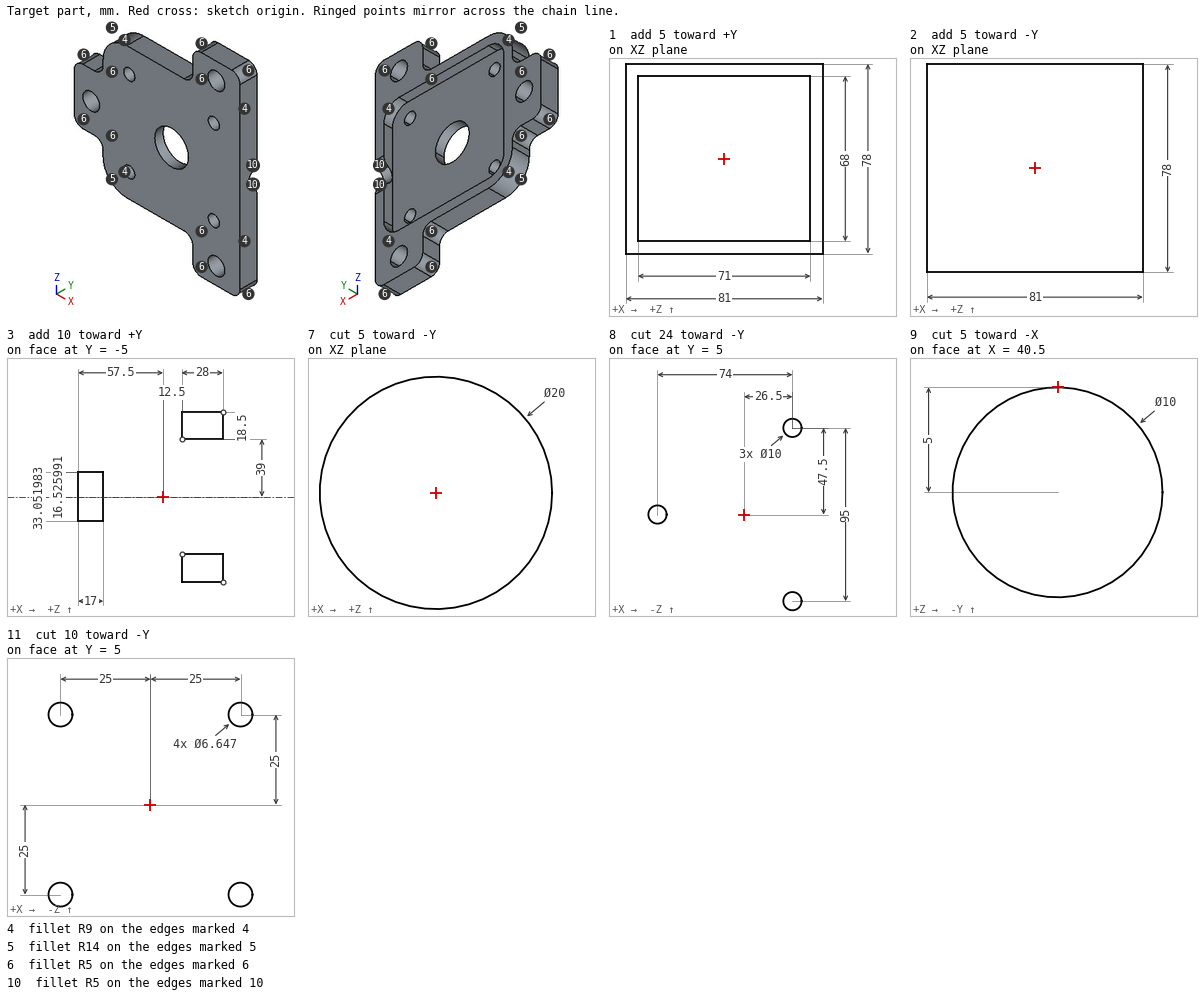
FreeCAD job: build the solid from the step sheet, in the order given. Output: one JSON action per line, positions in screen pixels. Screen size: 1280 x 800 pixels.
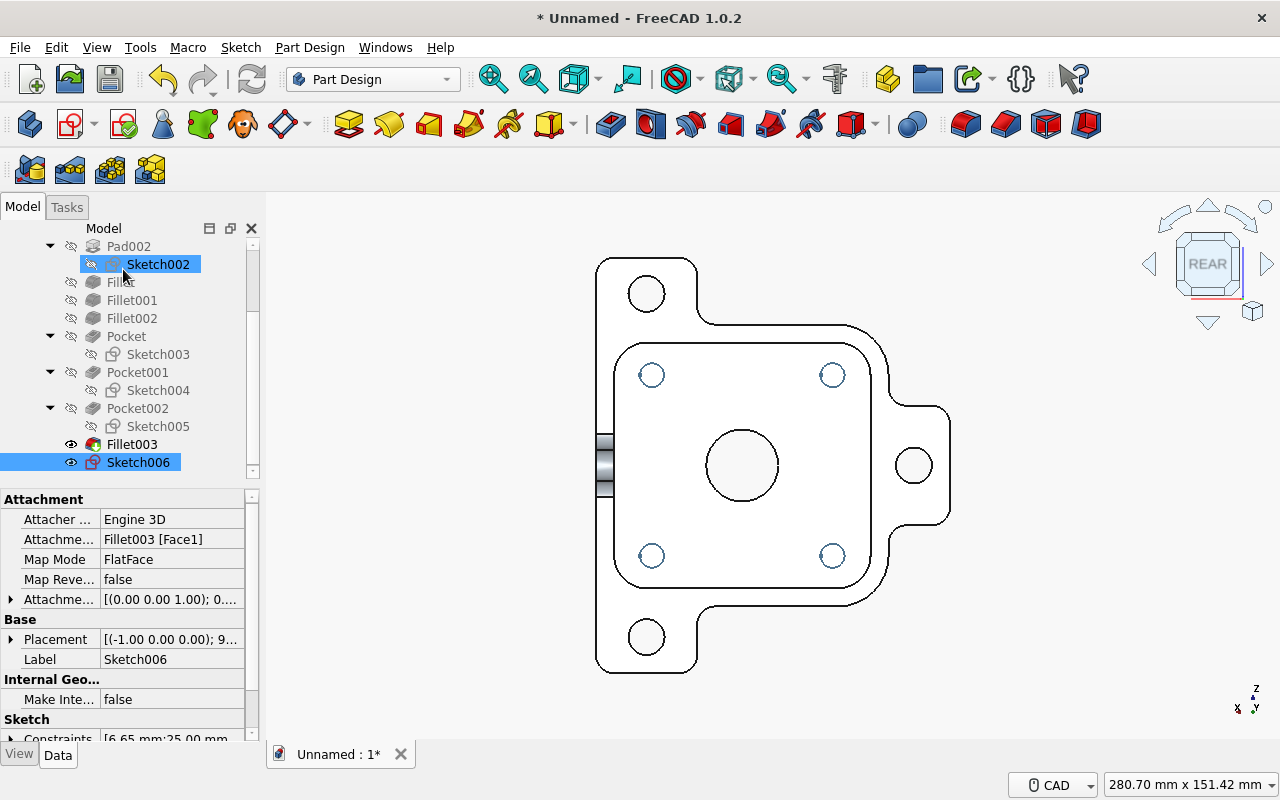
{"action": "left_click", "coordinate": [612, 124]}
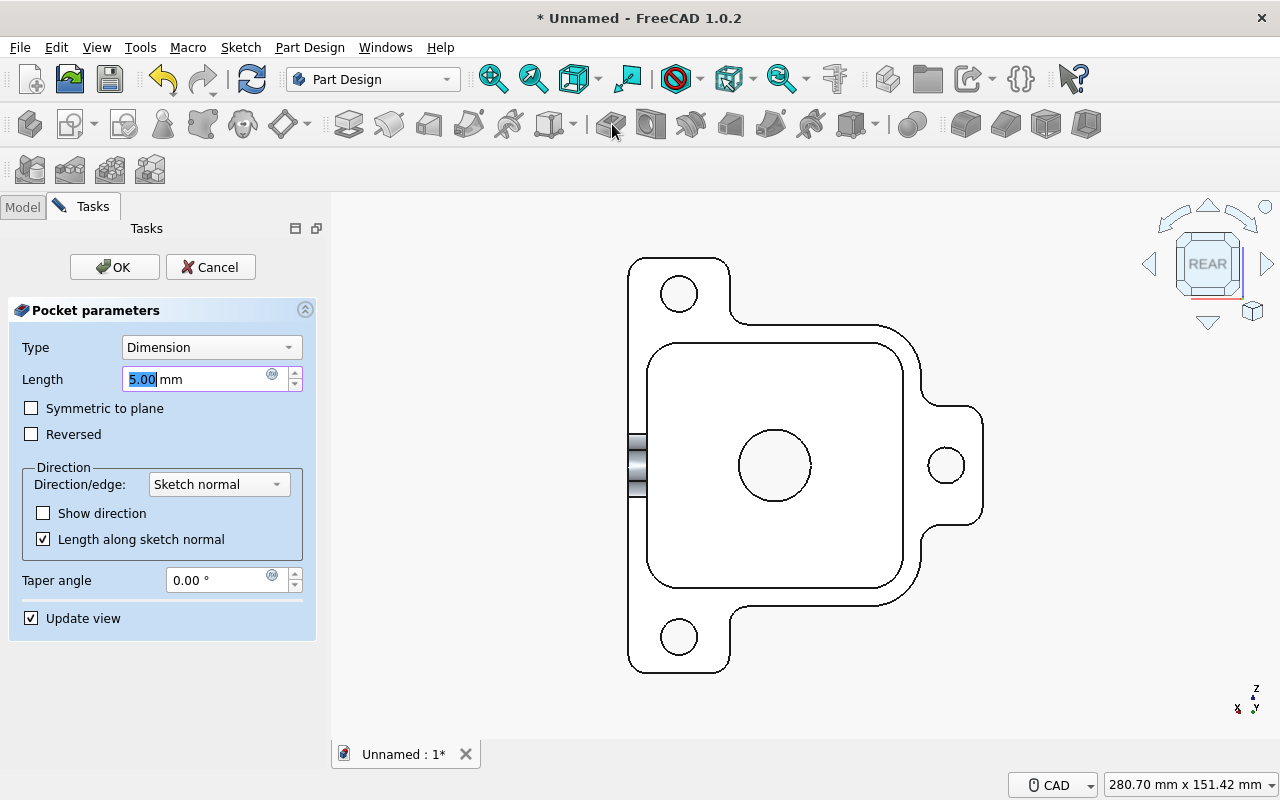
{"action": "type", "text": "10"}
{"action": "key", "text": "Tab"}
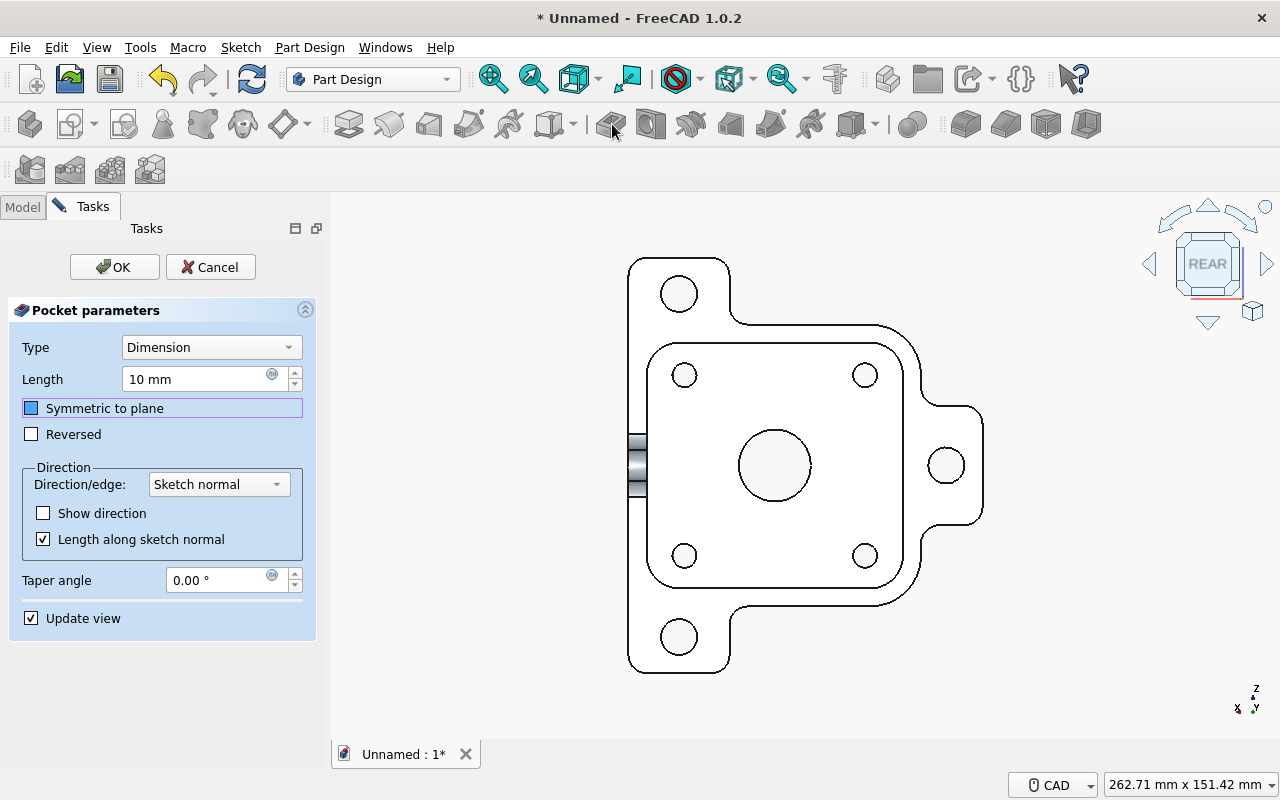
{"action": "left_click", "coordinate": [115, 267]}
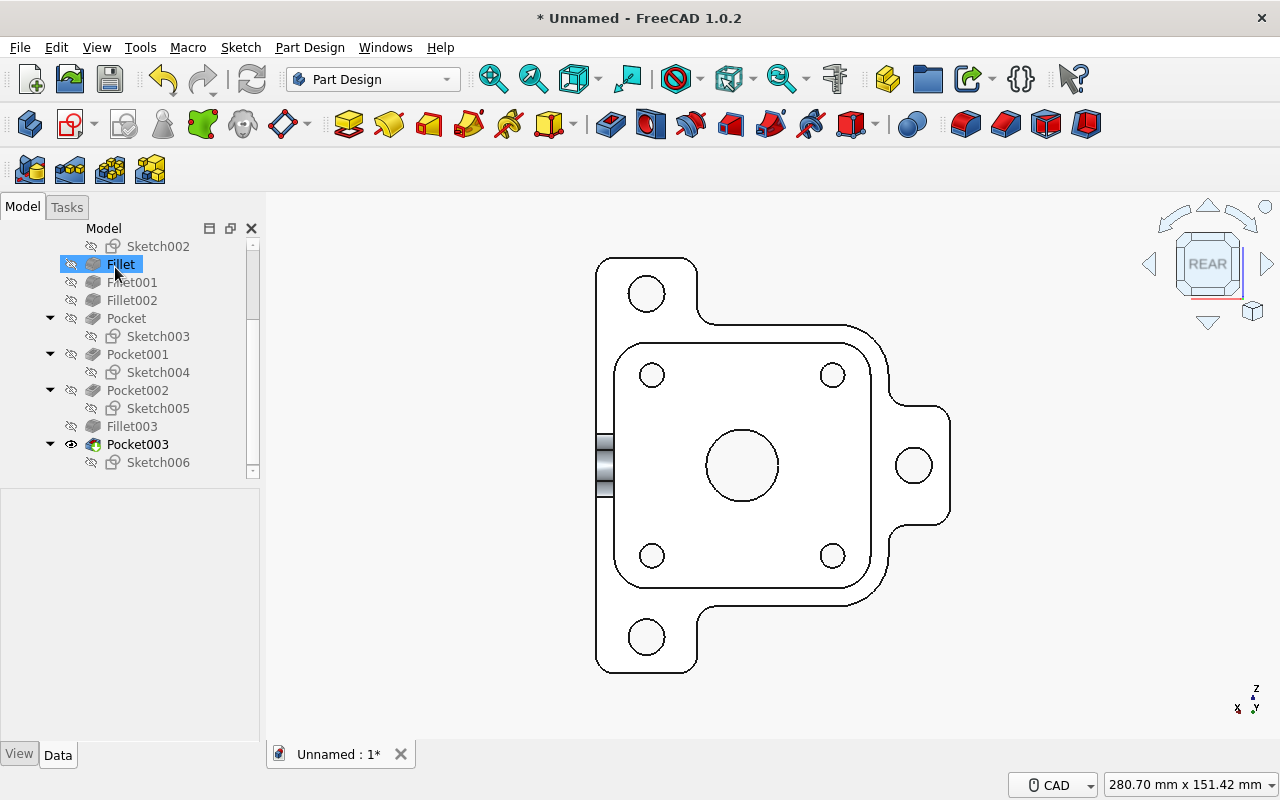
{"action": "key", "text": "0"}